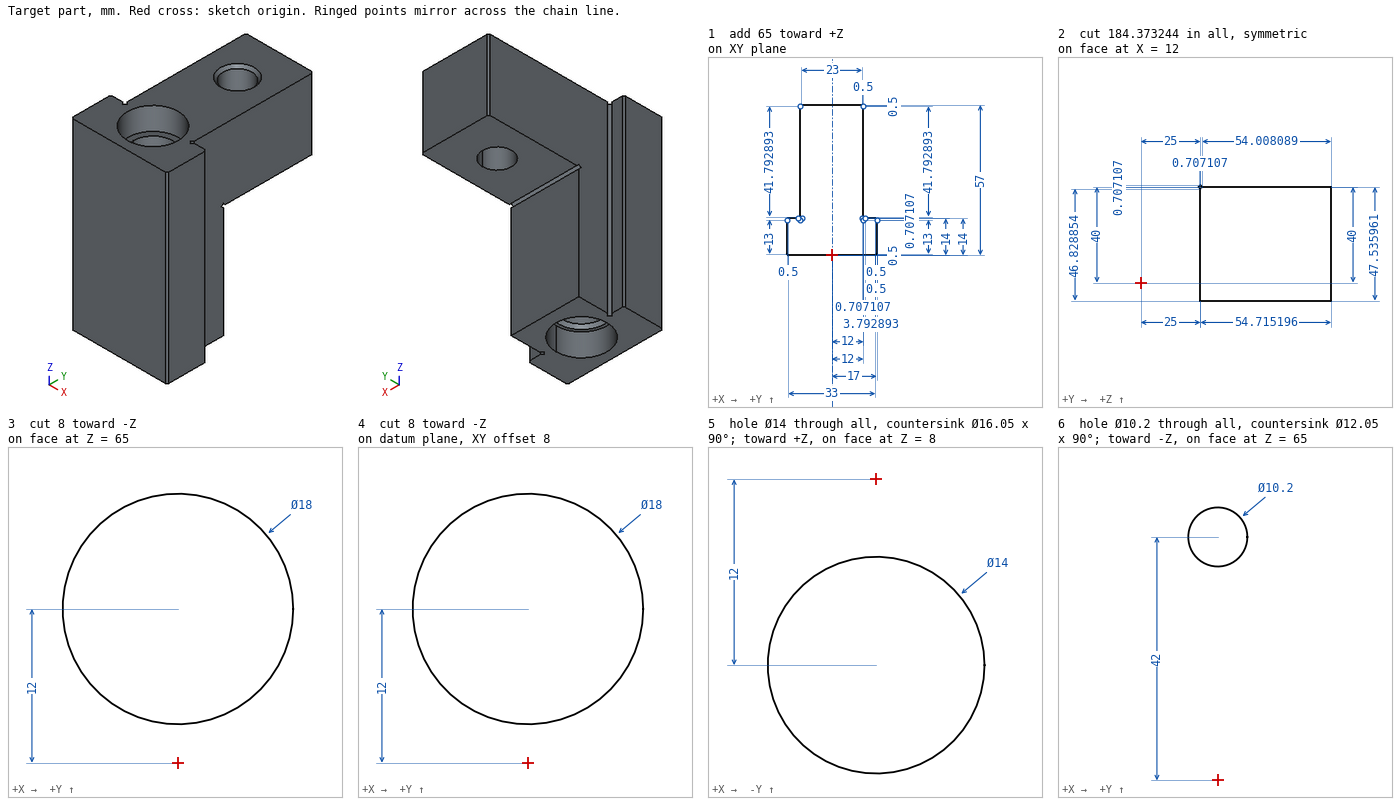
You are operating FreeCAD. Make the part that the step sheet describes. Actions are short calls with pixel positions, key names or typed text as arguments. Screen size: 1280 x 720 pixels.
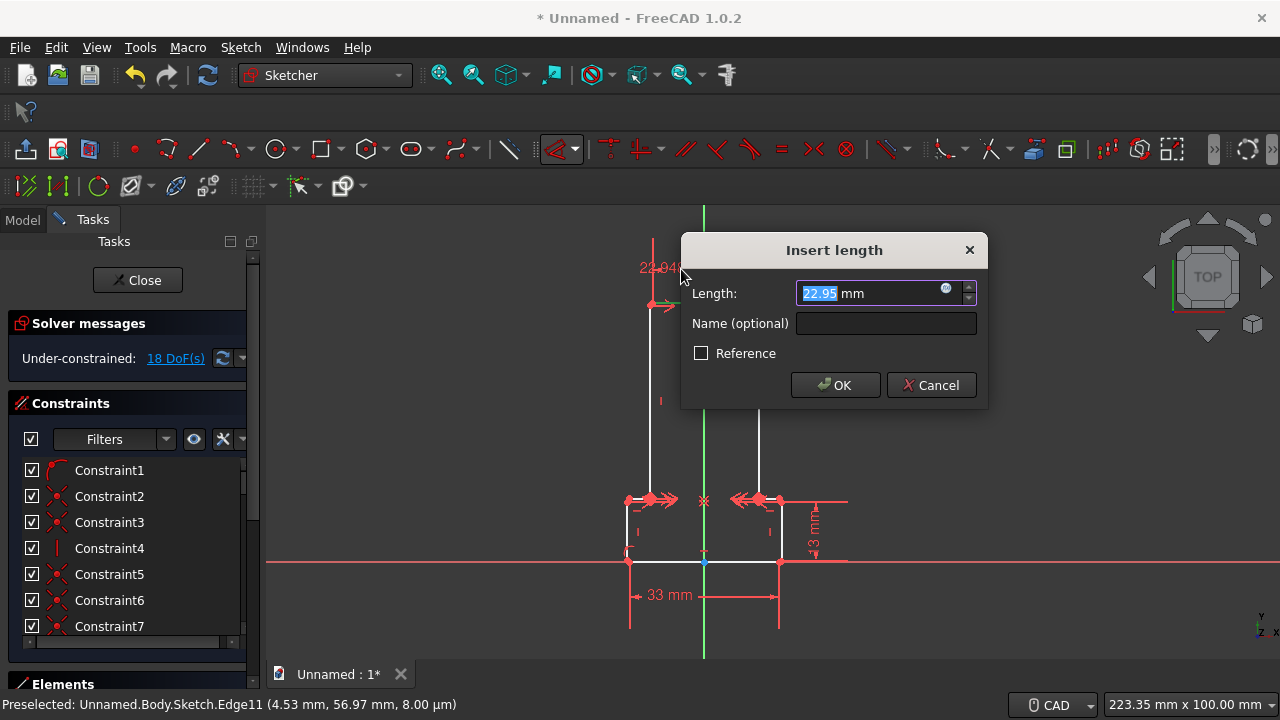
text(23)
key(Return)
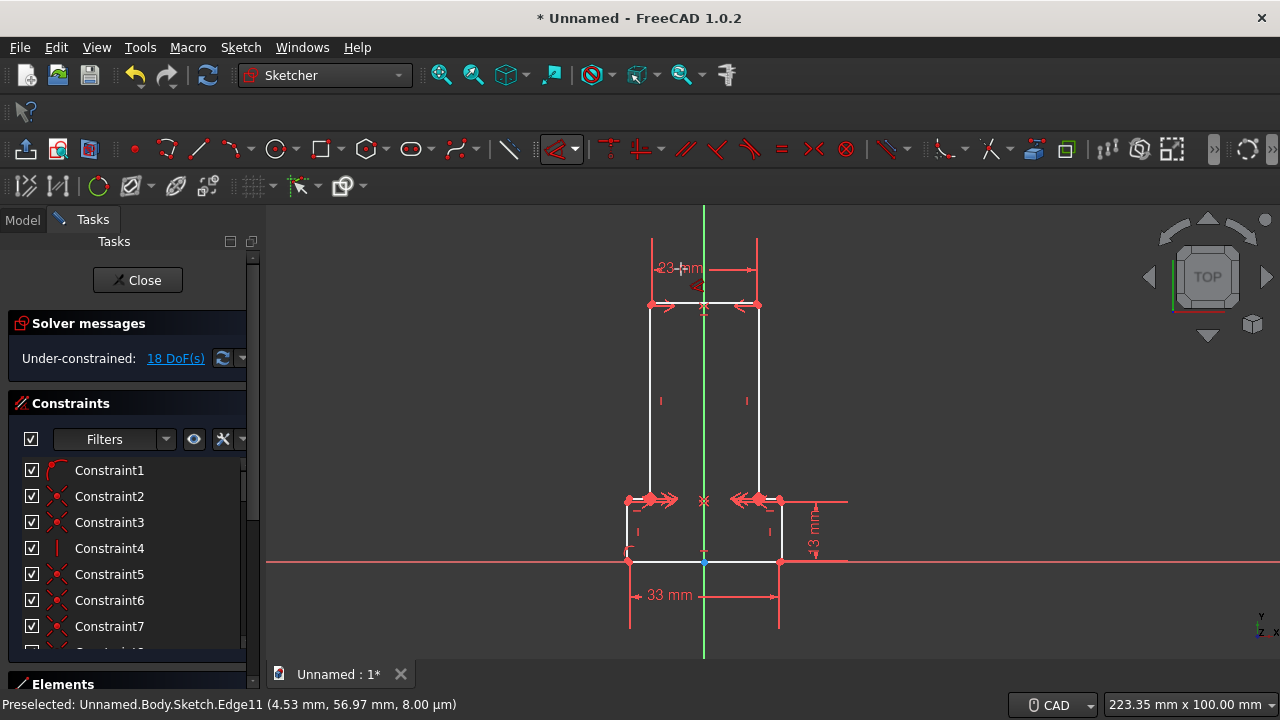
click(627, 519)
click(593, 531)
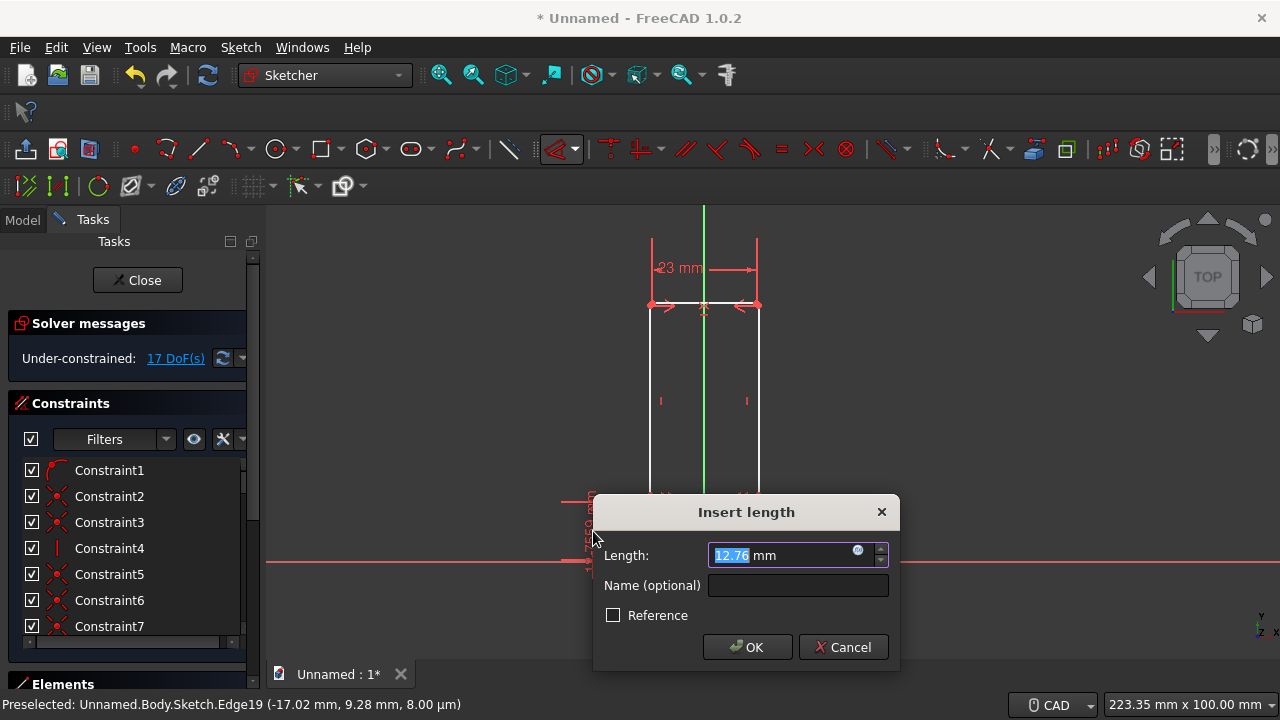
text(13)
key(Return)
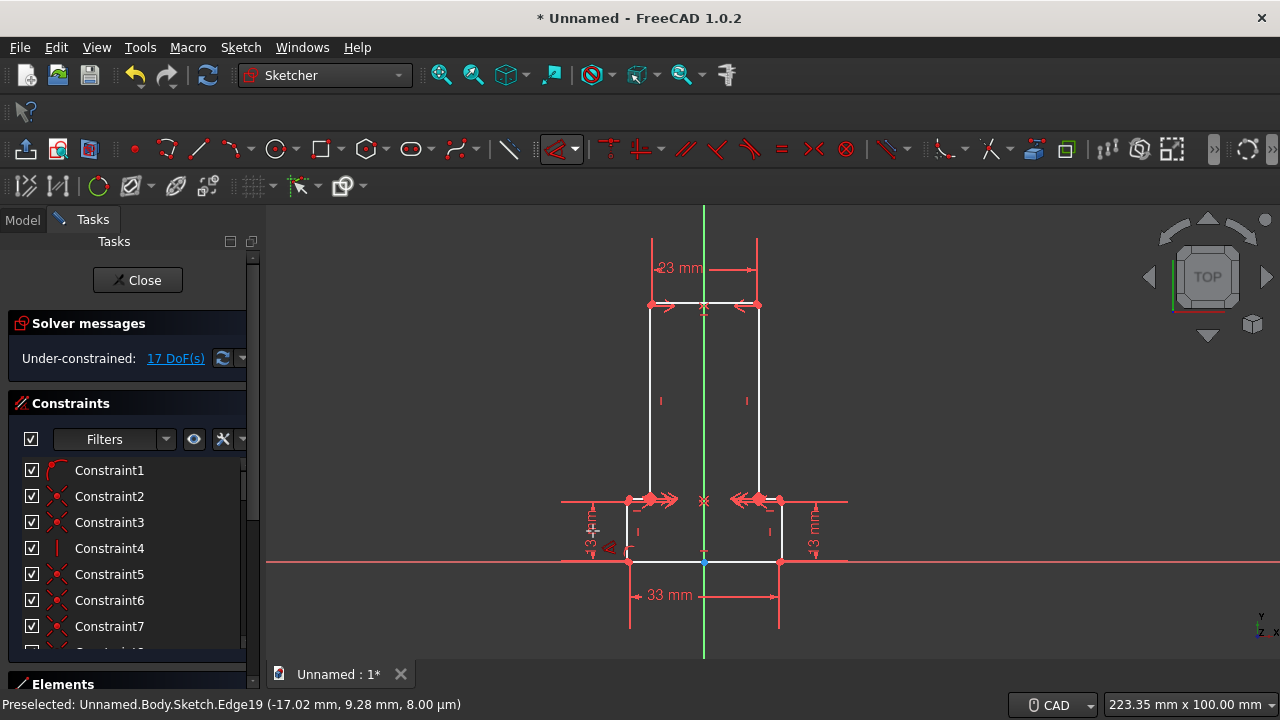
scroll(782, 561, up, 8)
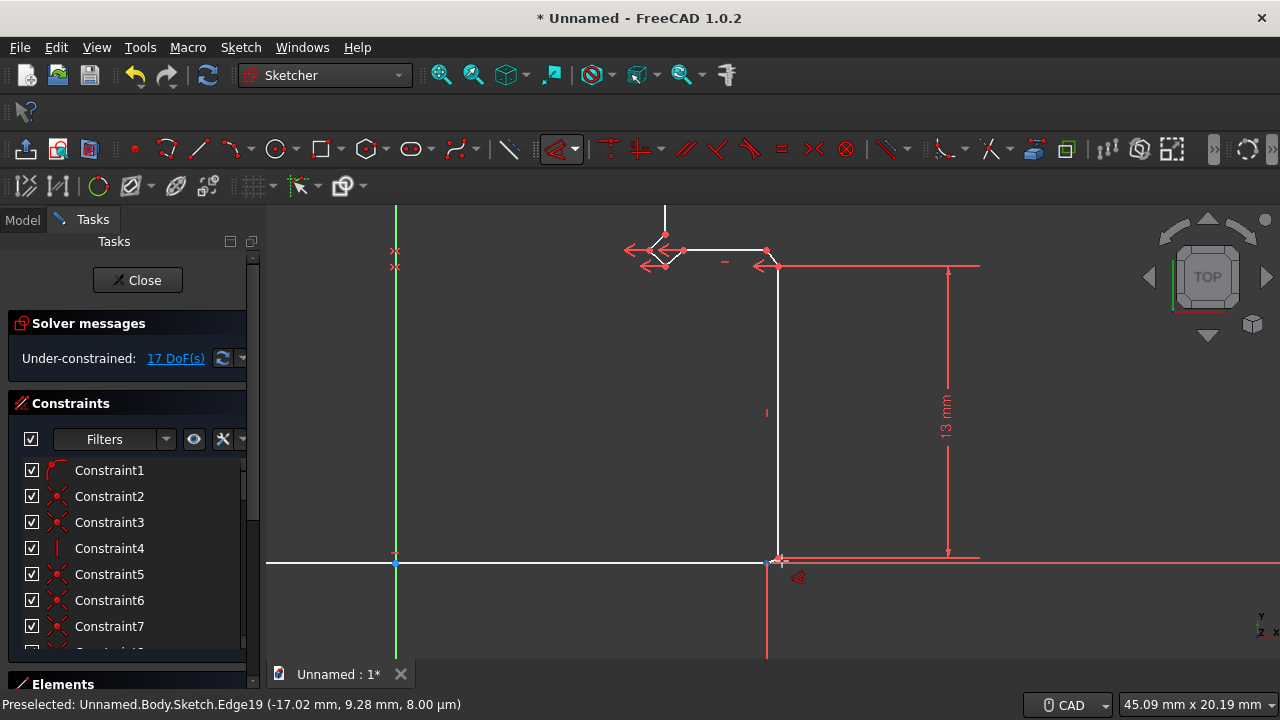
click(778, 558)
click(587, 597)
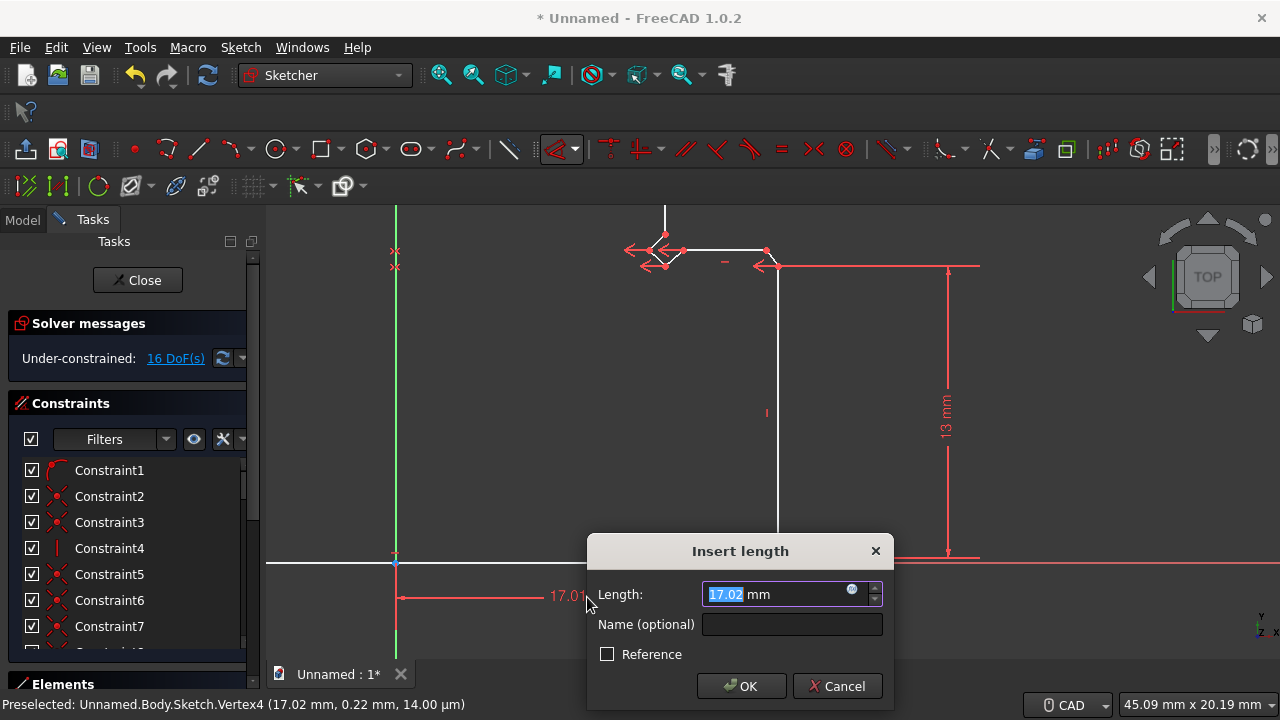
text(17)
key(Return)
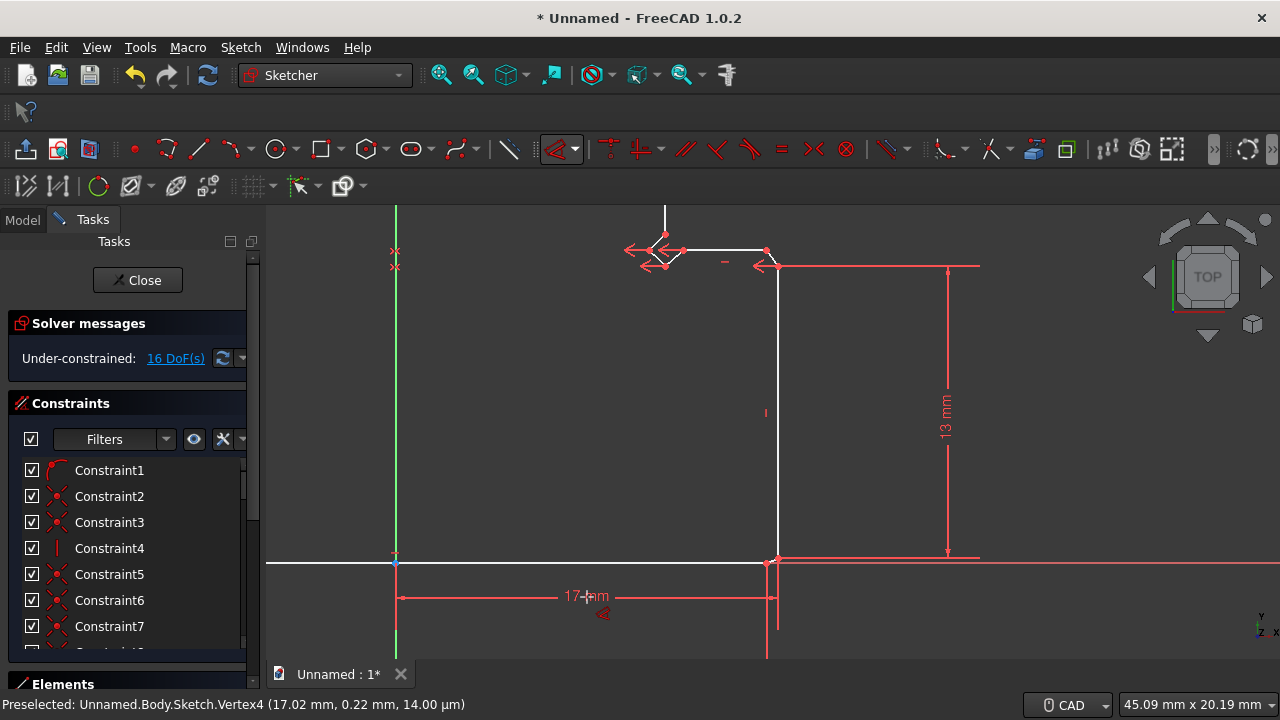
click(767, 250)
click(801, 407)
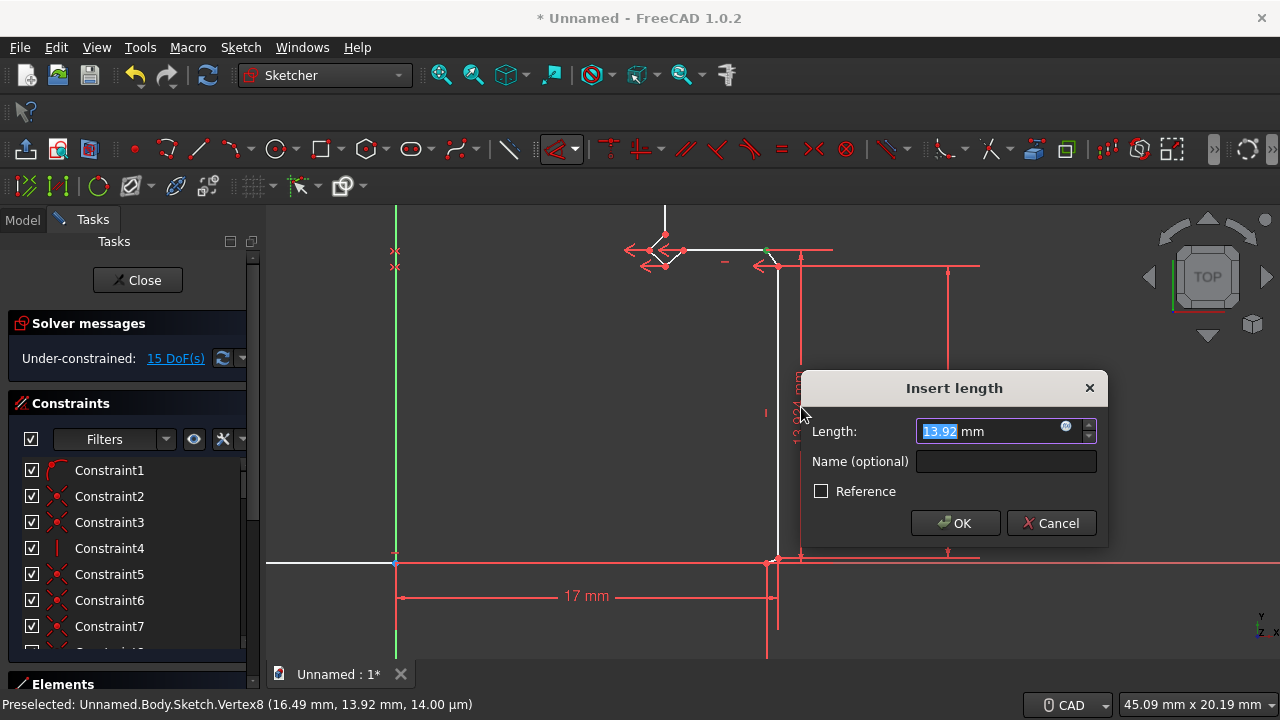
text(14)
key(Return)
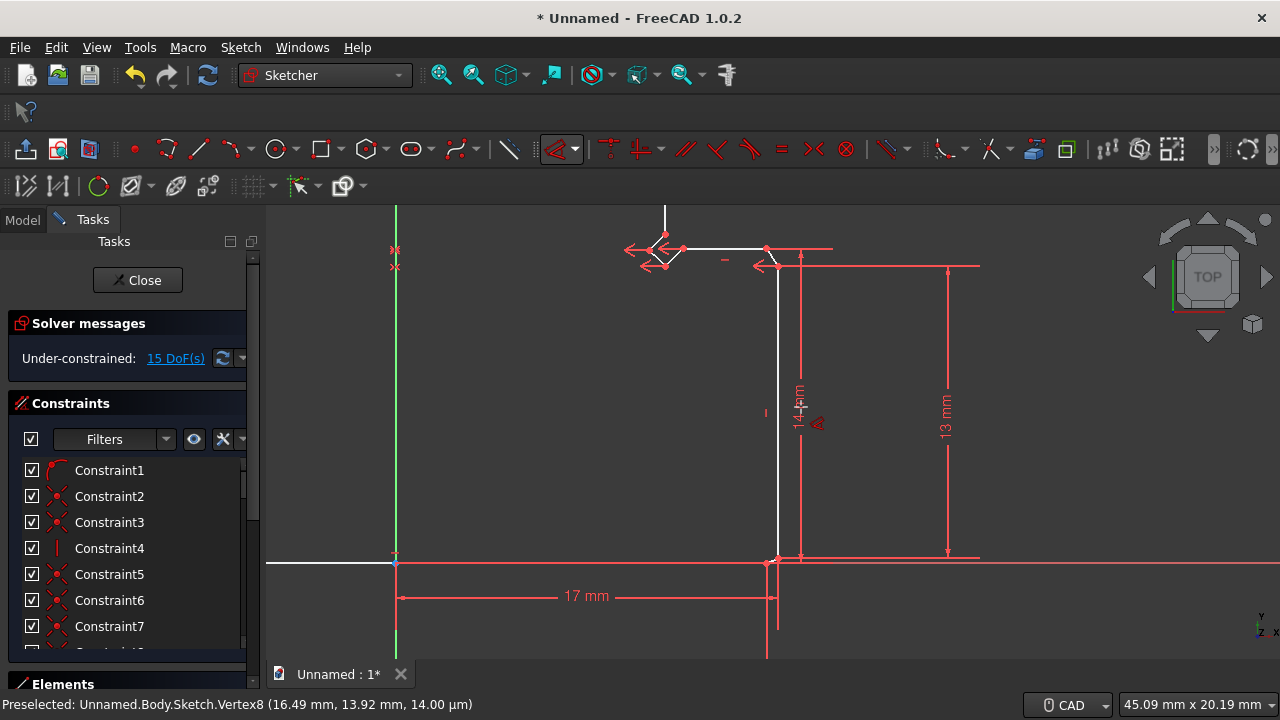
click(665, 266)
click(469, 597)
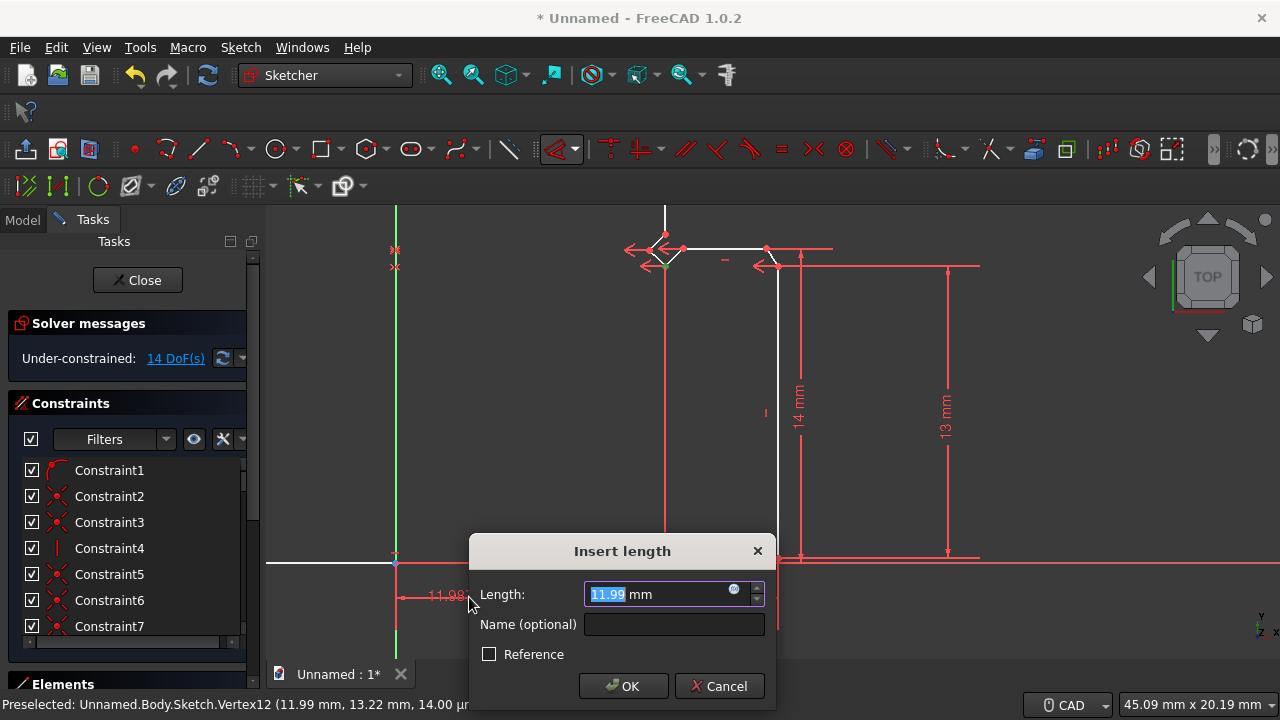
text(12)
key(Return)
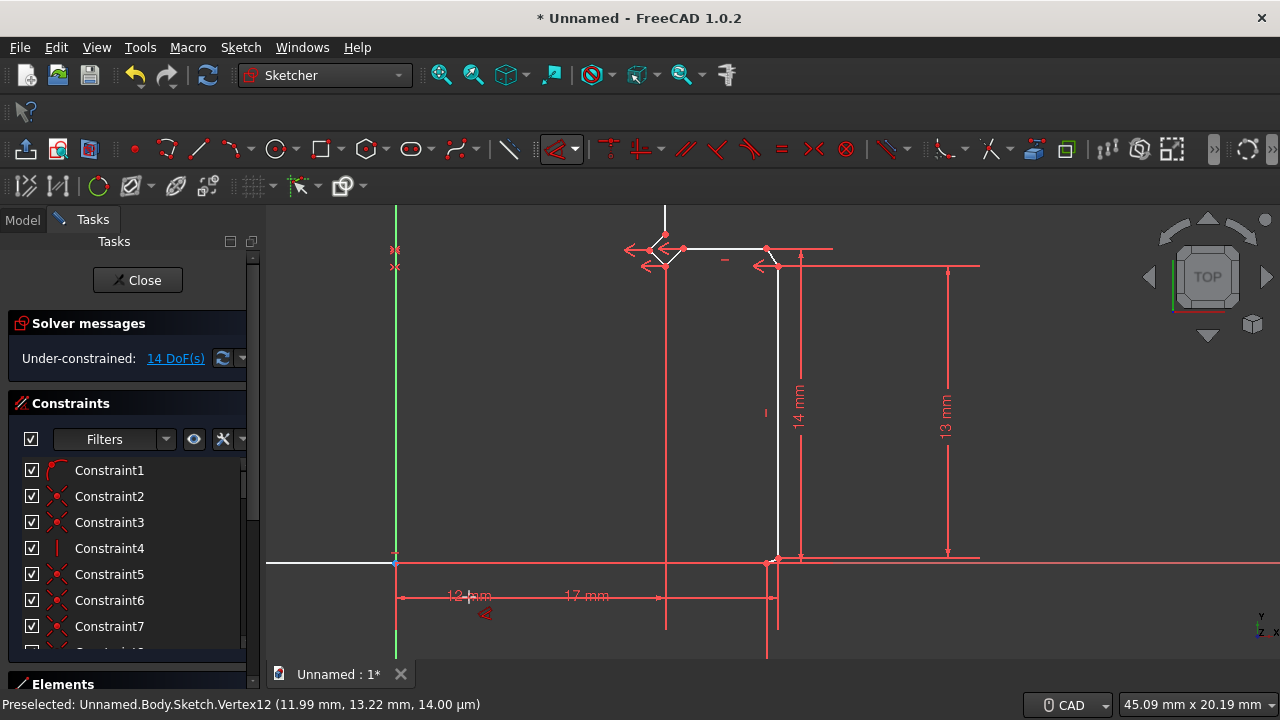
click(649, 250)
click(683, 407)